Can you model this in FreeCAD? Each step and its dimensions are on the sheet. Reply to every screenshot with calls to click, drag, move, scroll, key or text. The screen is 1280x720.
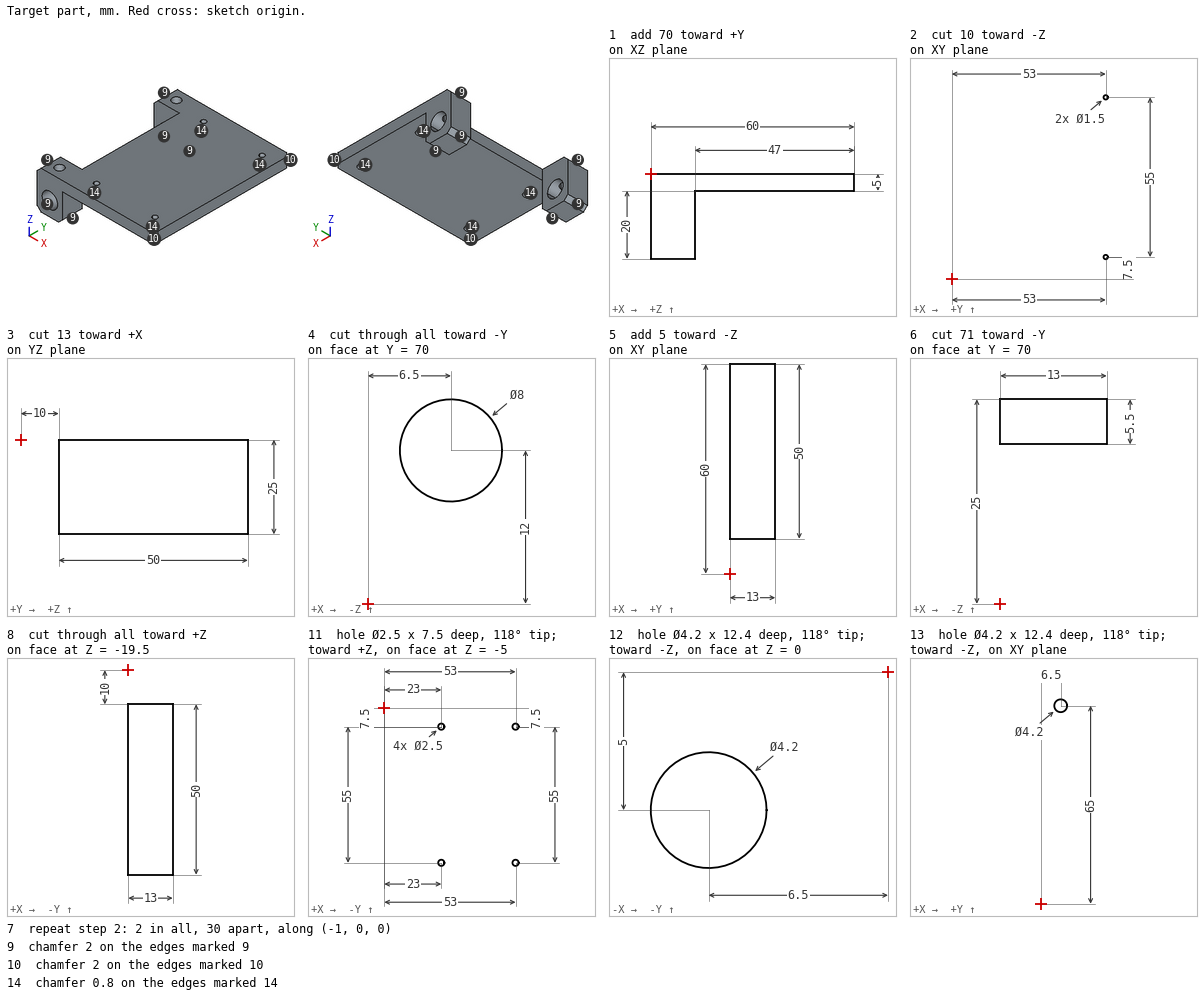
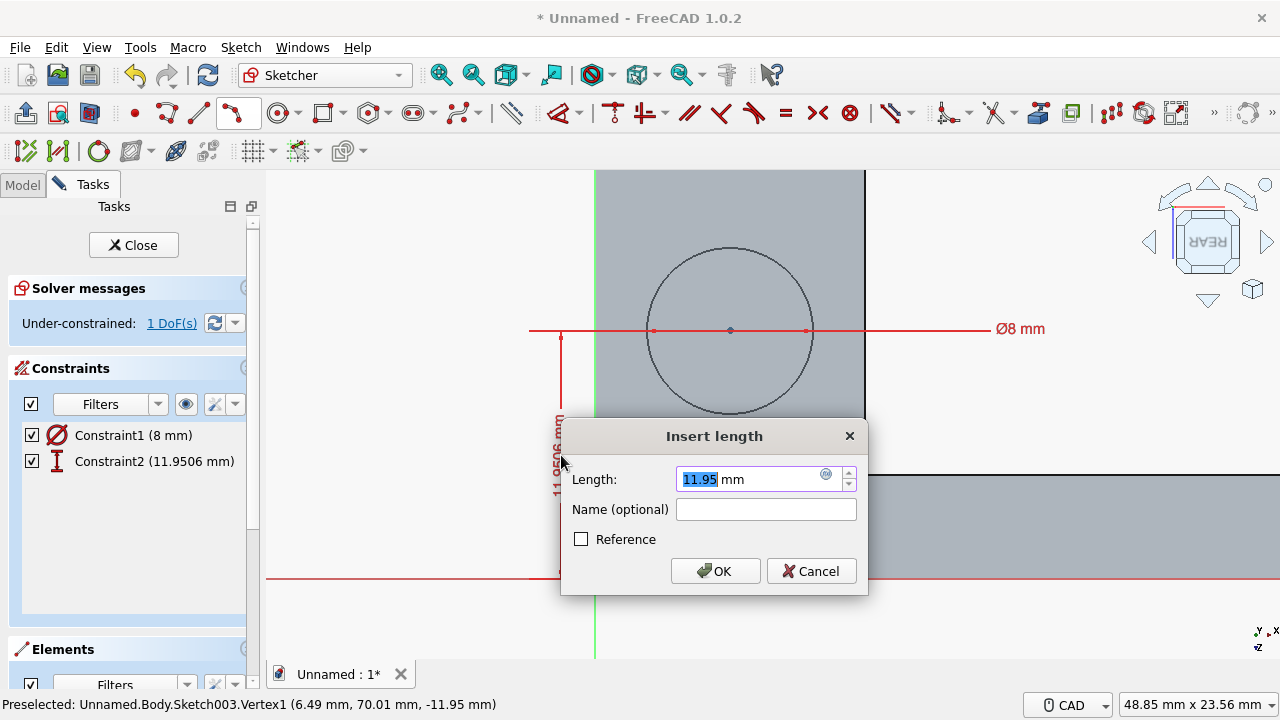
text(12)
key(Return)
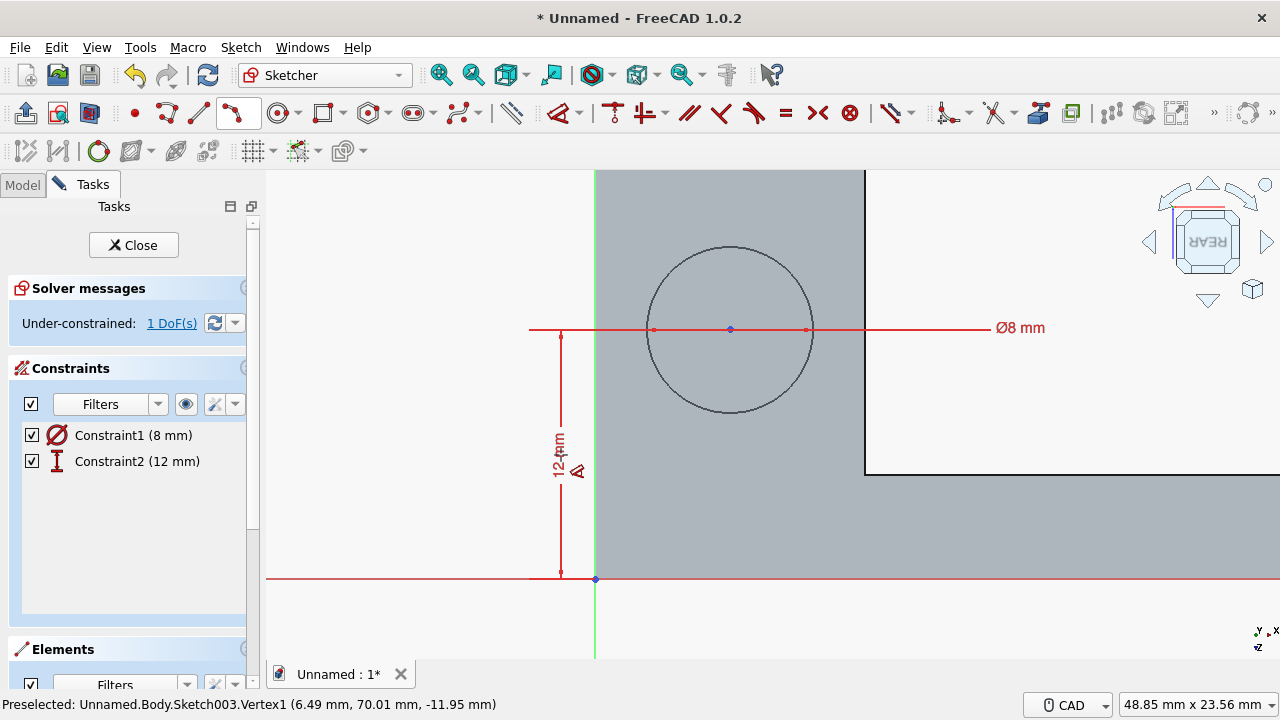
click(730, 330)
click(663, 613)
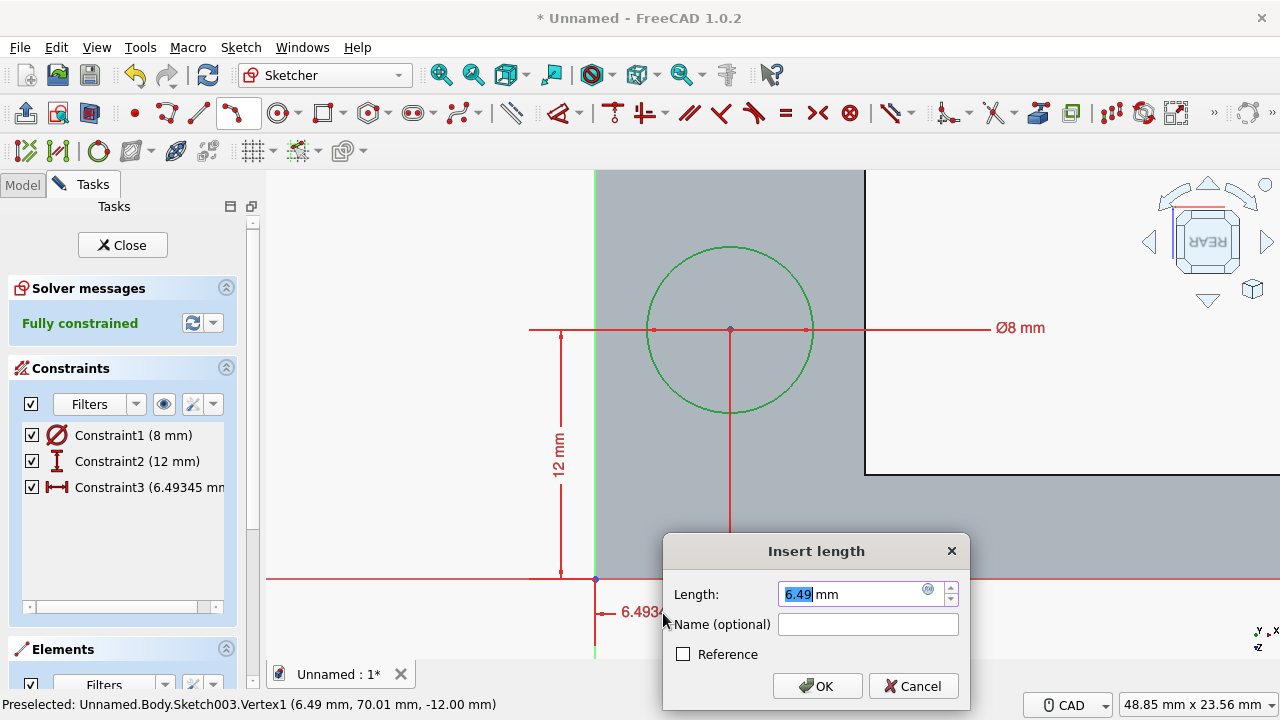
text(6.5)
key(Return)
key(Escape)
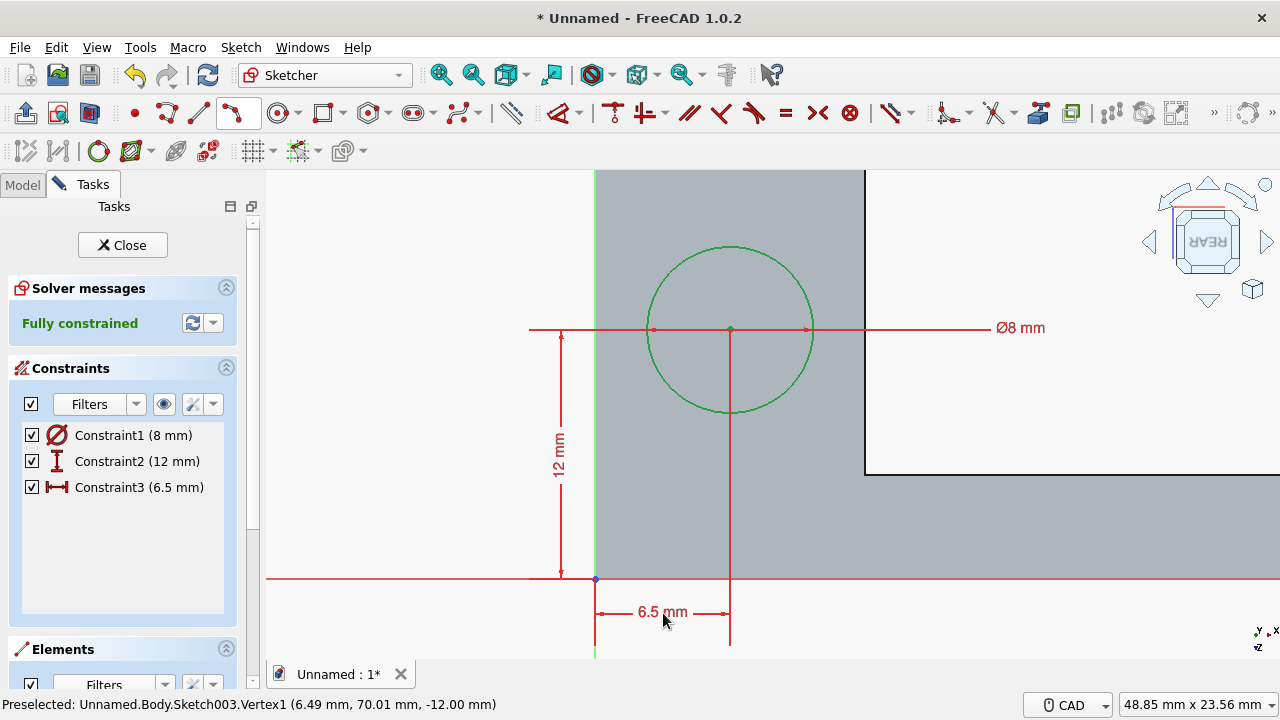
click(123, 245)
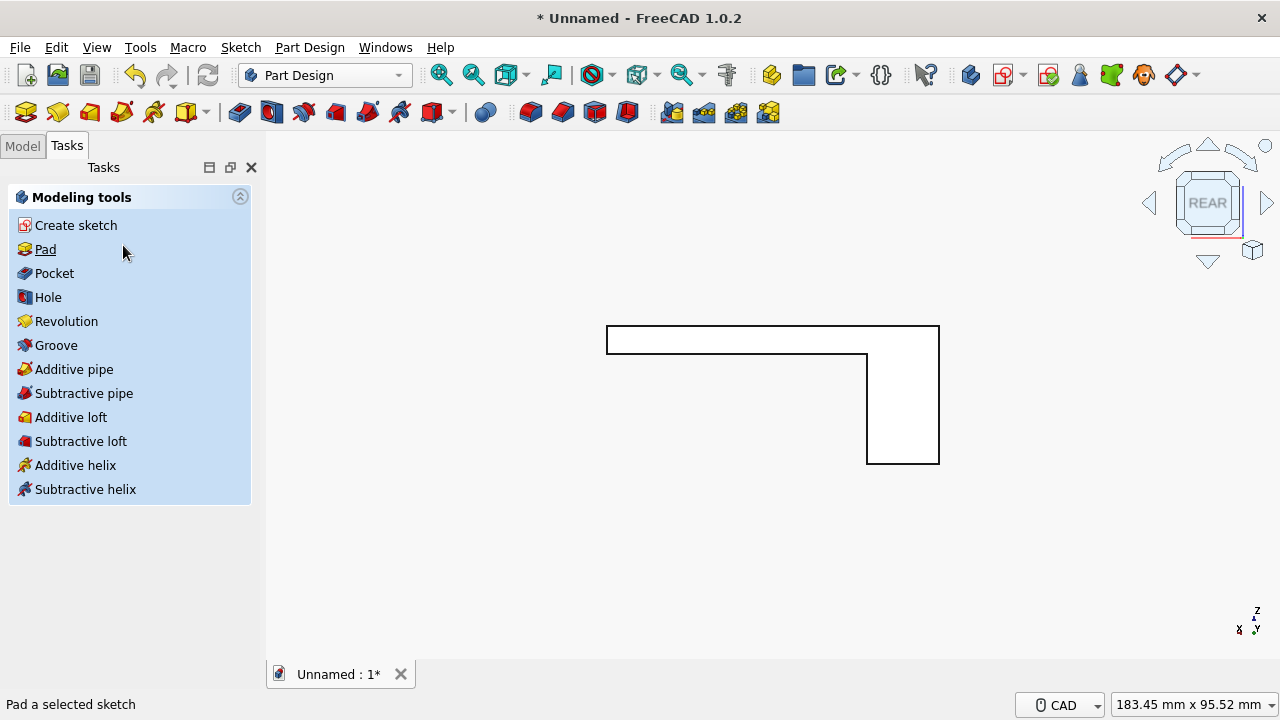
click(240, 112)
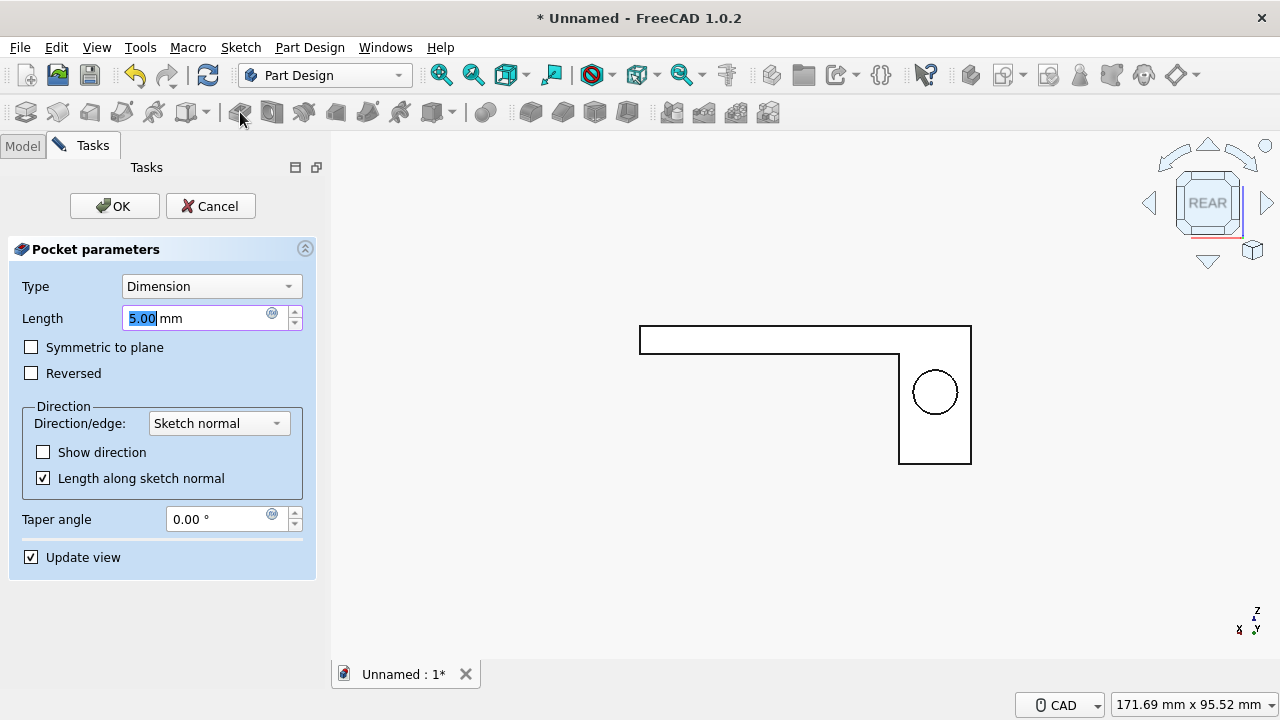
click(212, 286)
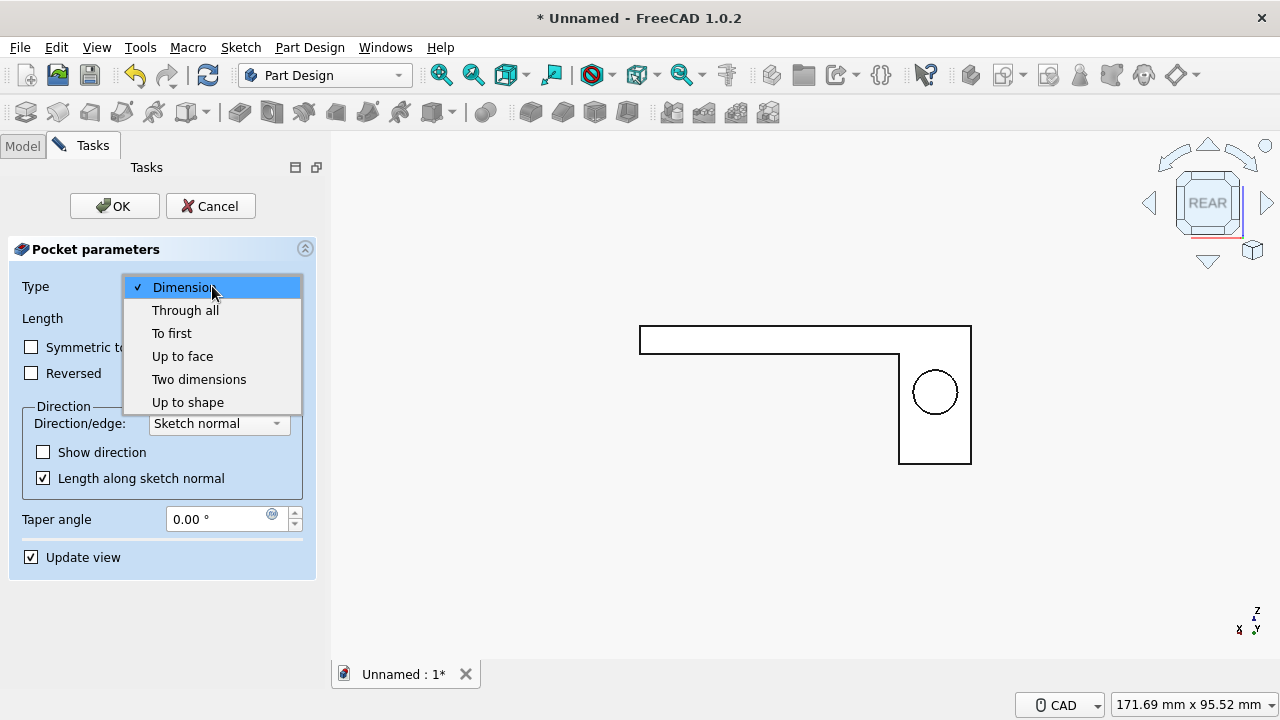
click(212, 310)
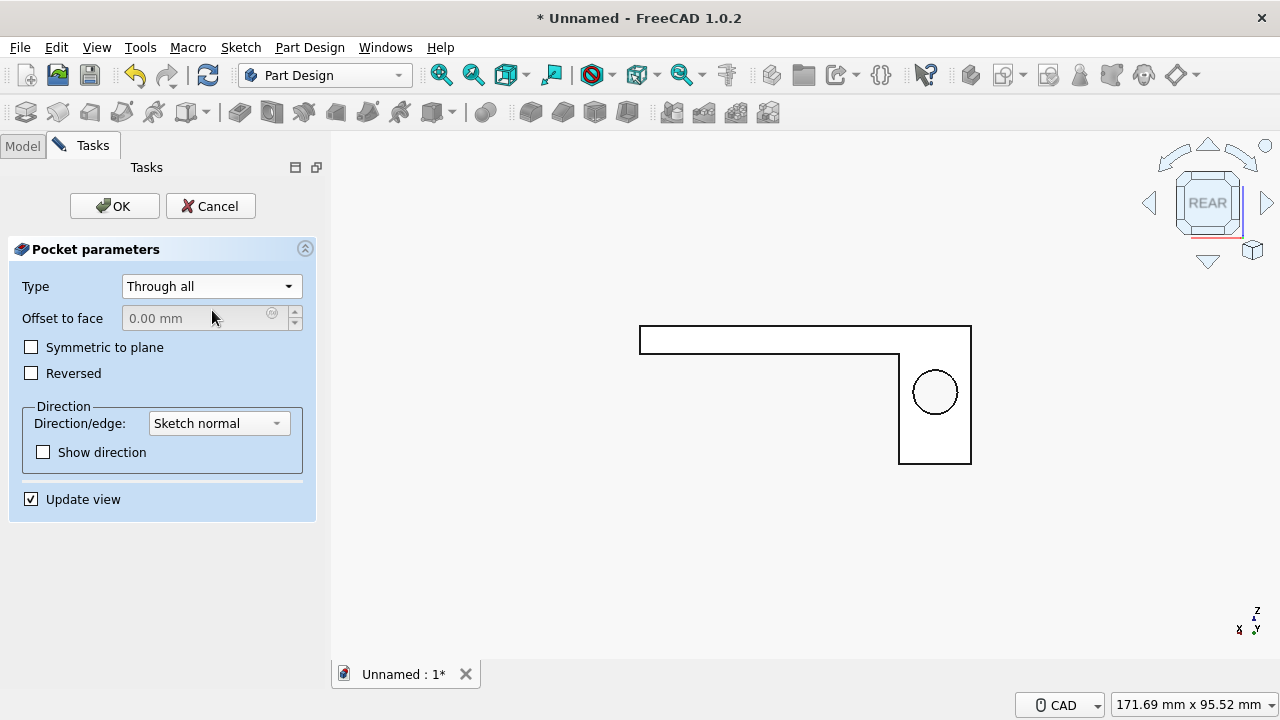
click(115, 206)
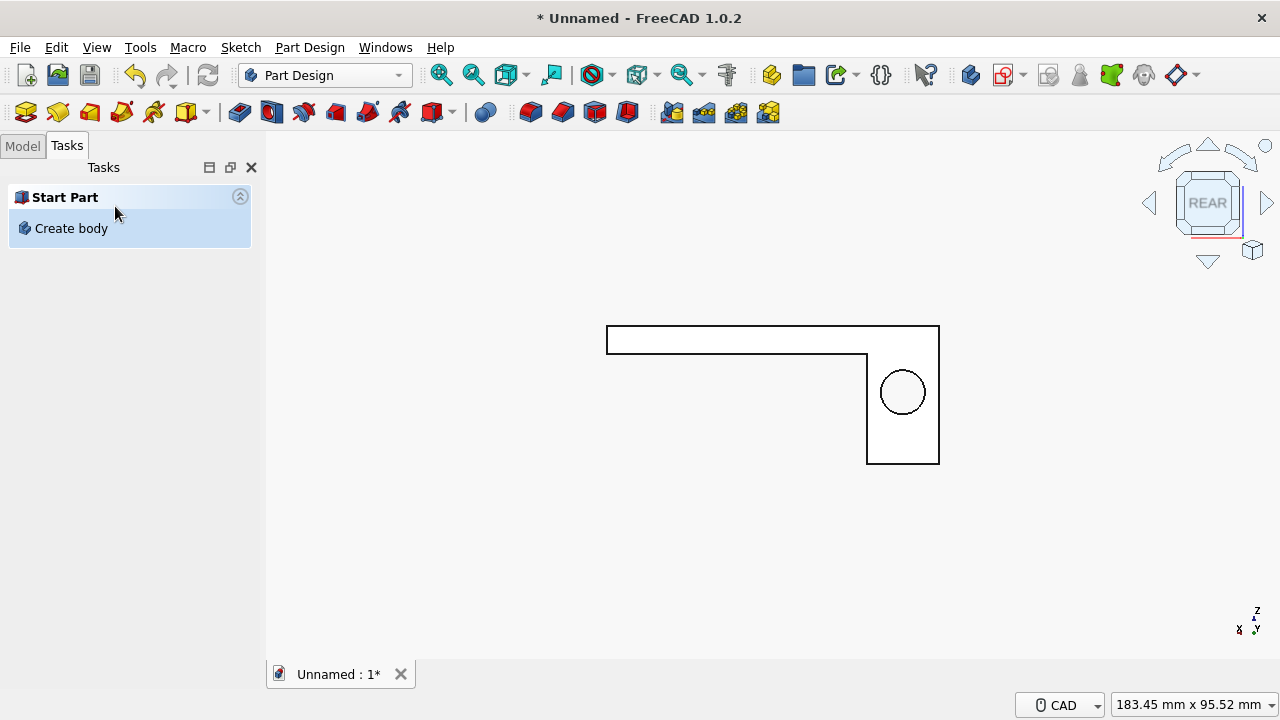
key(v)
key(f)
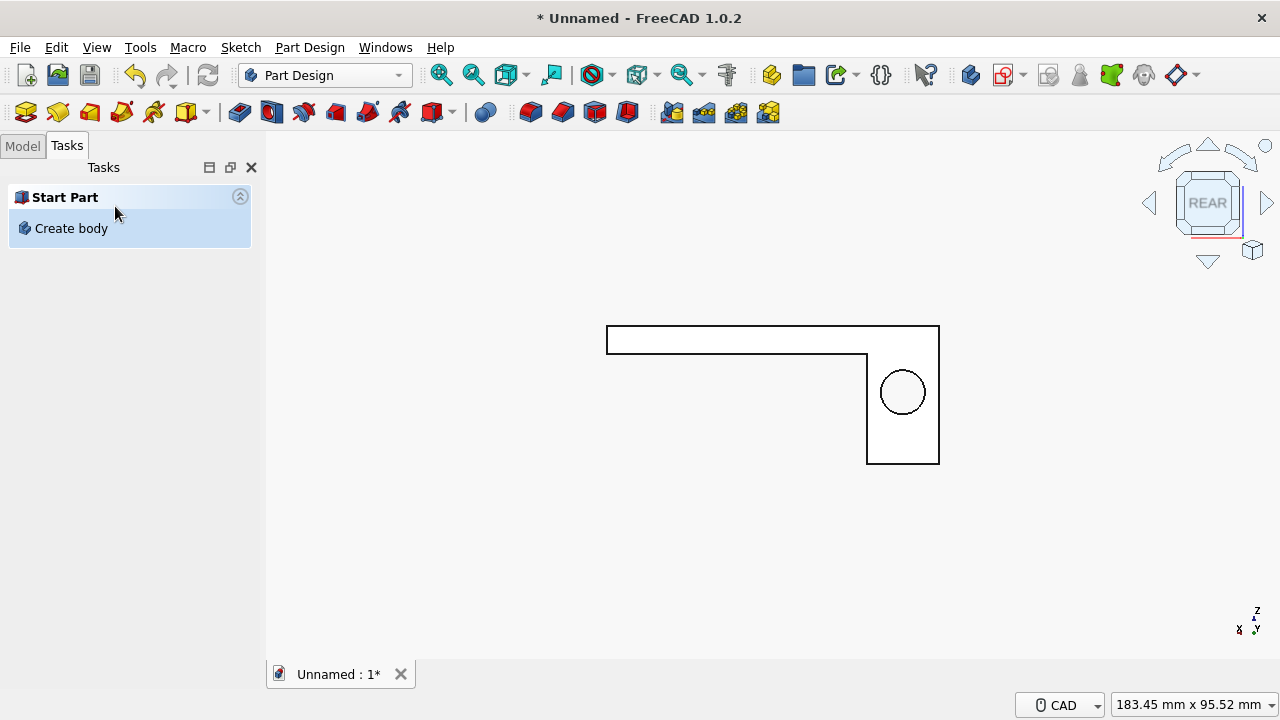
click(1004, 76)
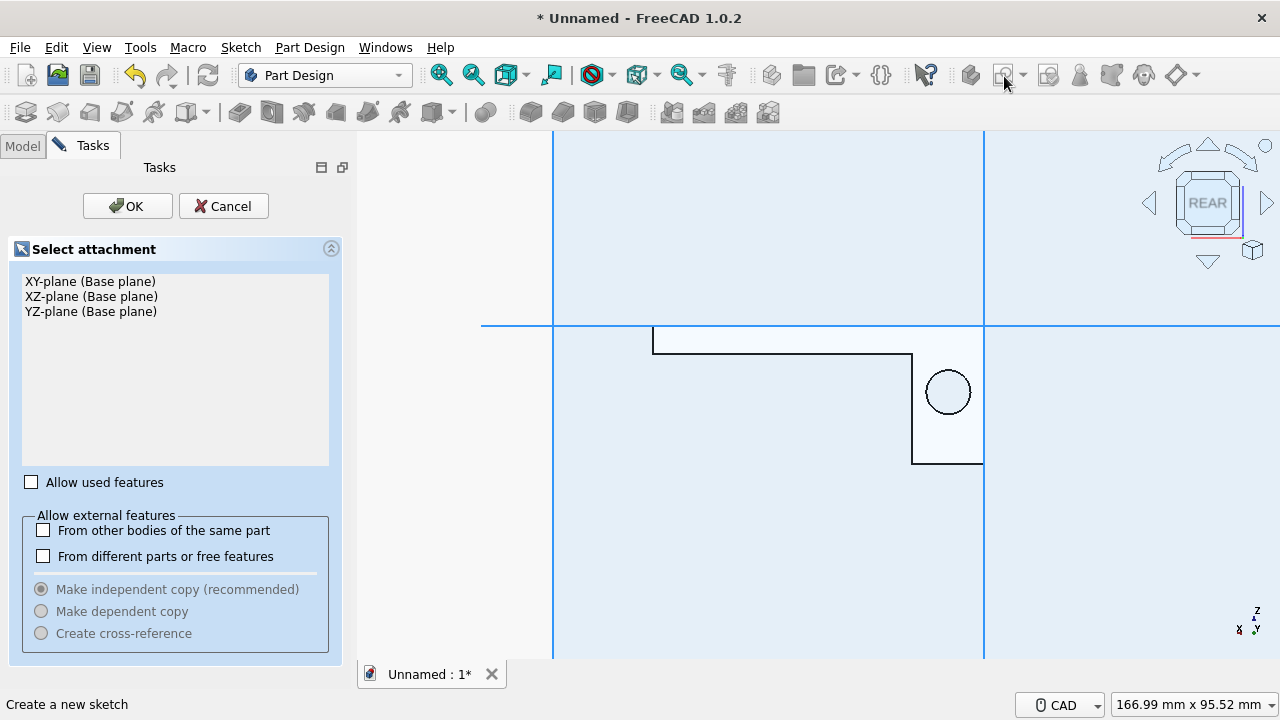
click(82, 282)